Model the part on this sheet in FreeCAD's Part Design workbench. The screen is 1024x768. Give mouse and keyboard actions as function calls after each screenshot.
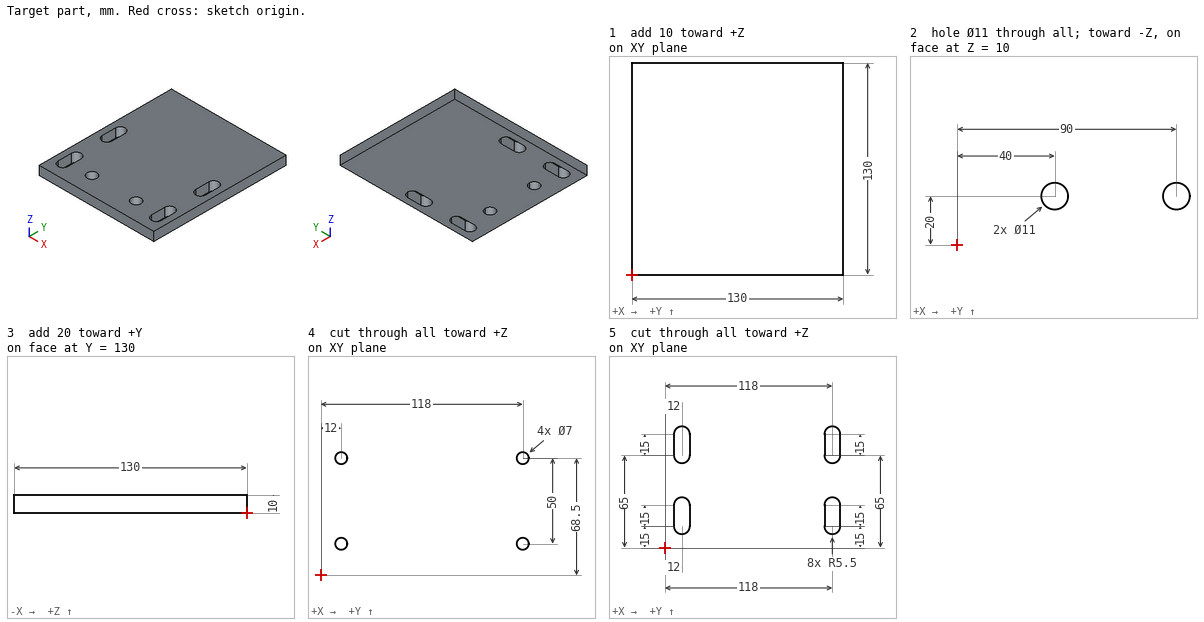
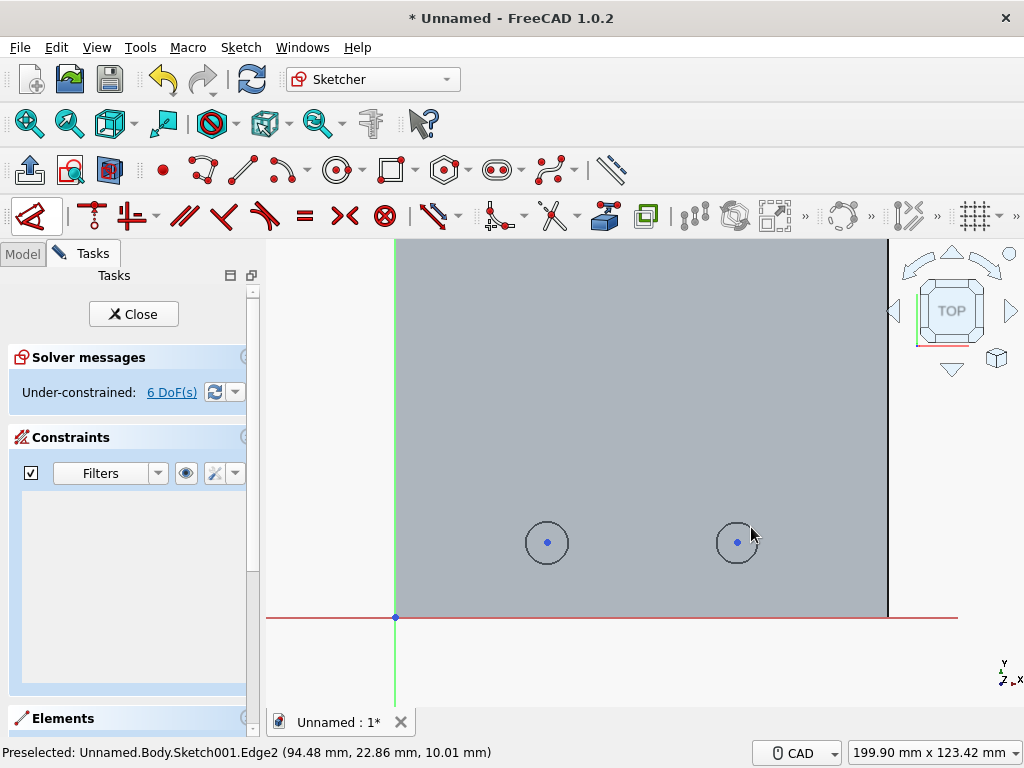
click(562, 528)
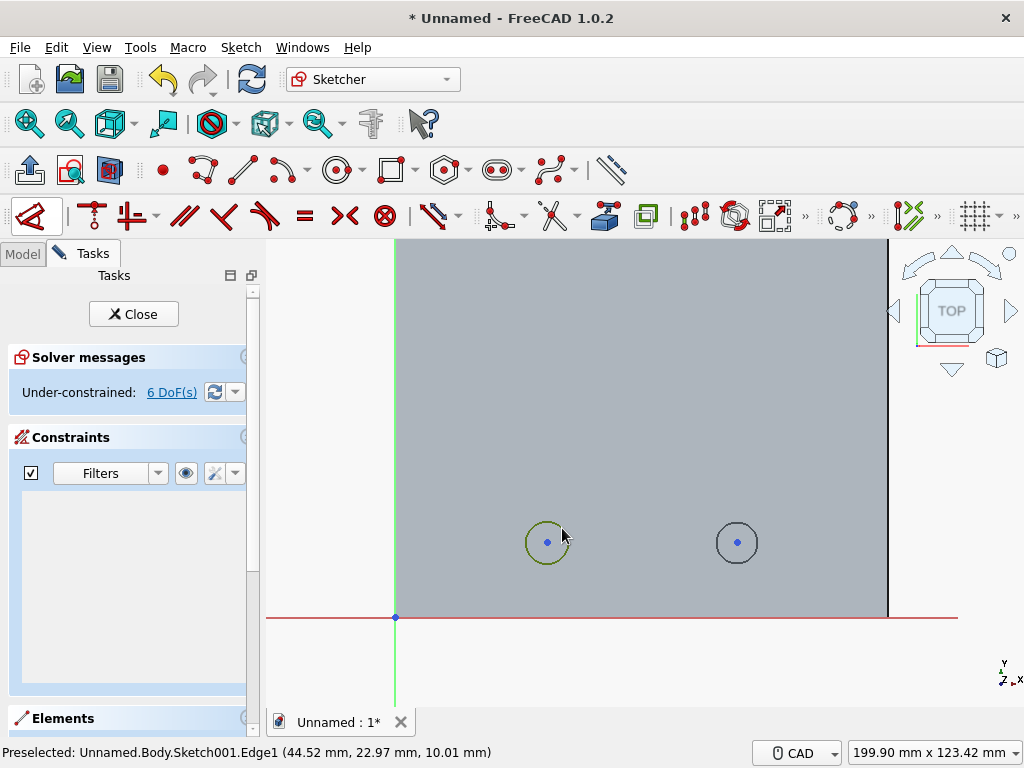
click(751, 528)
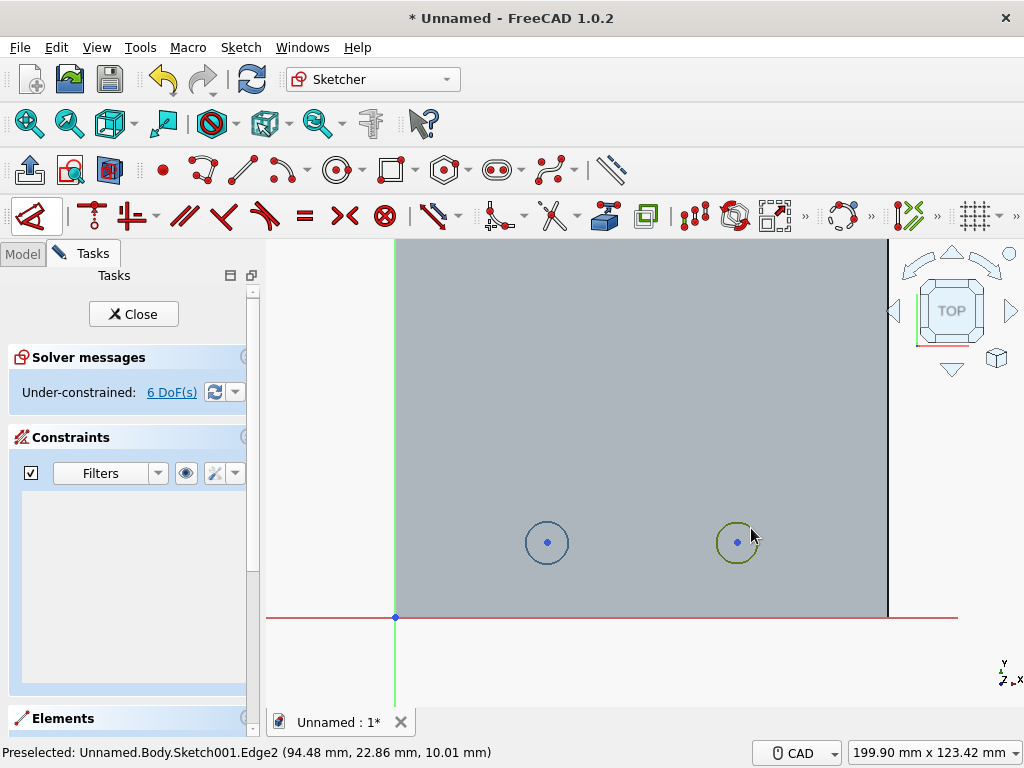
click(306, 216)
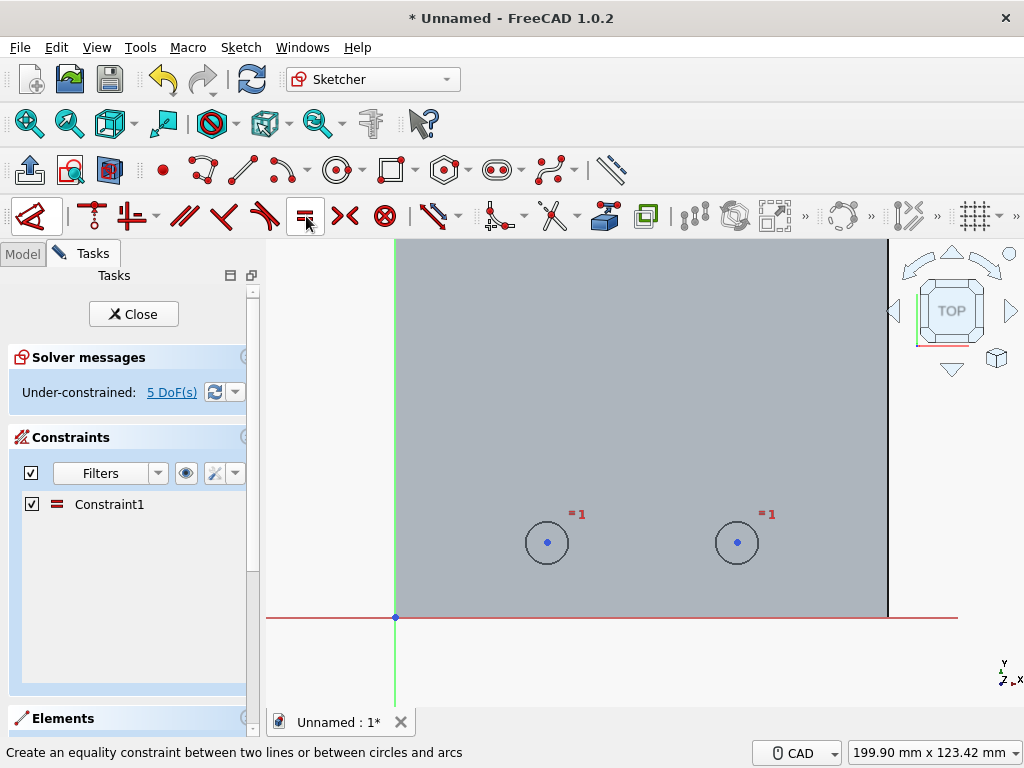
click(547, 543)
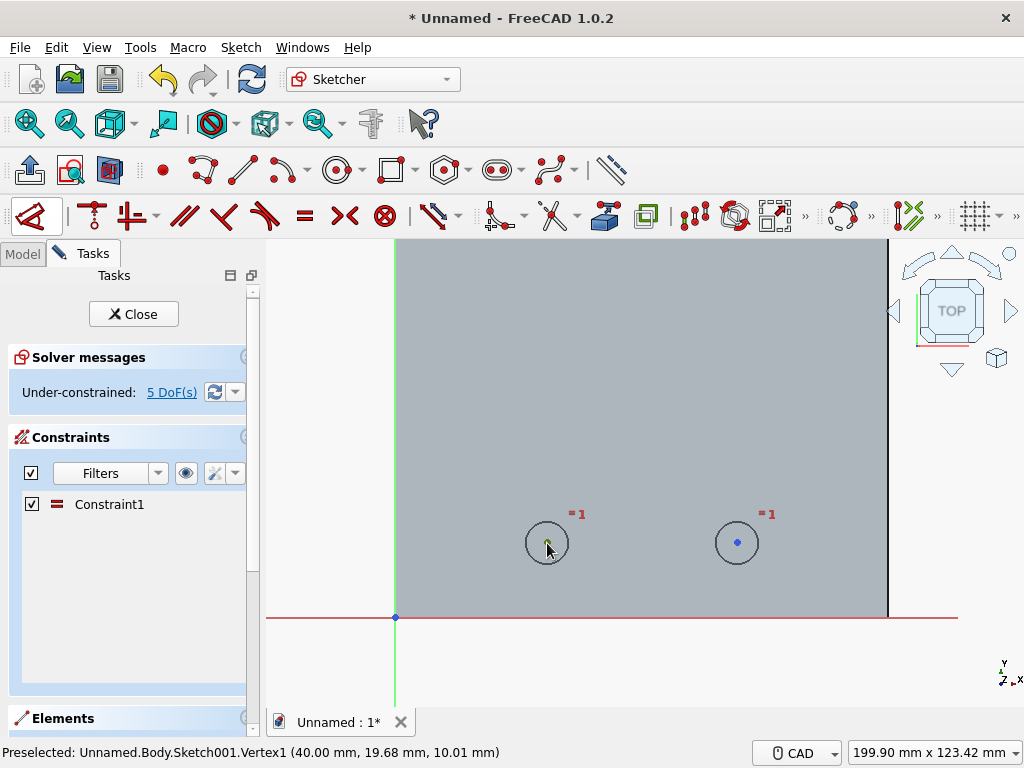
click(737, 543)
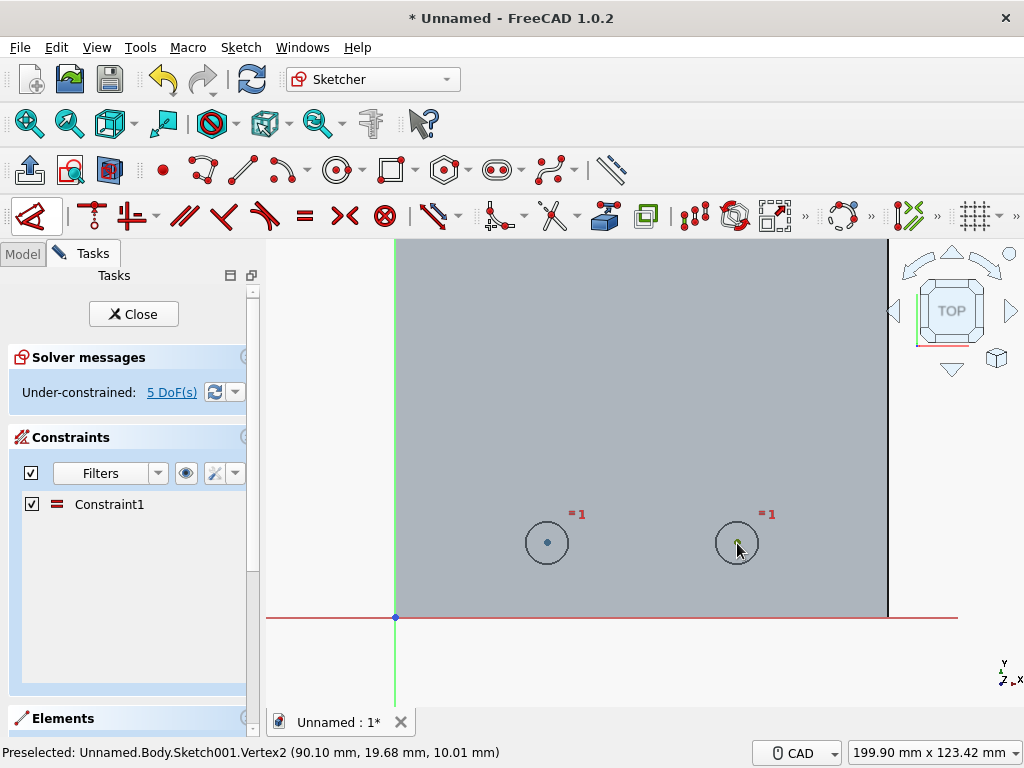
key(h)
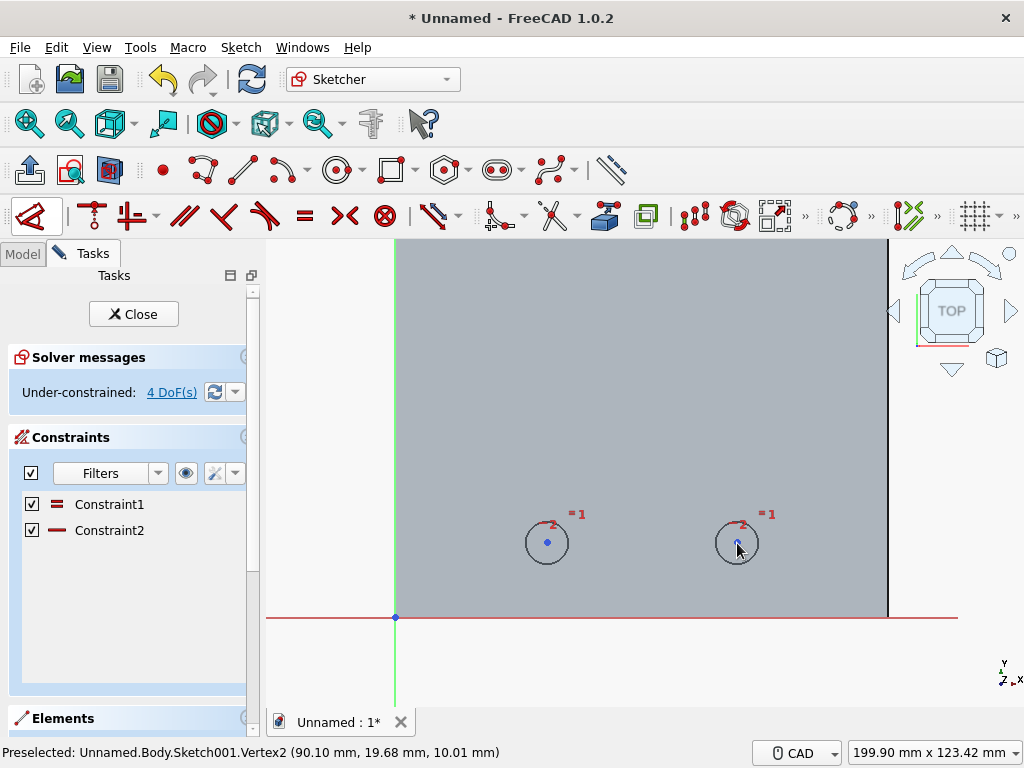
click(562, 528)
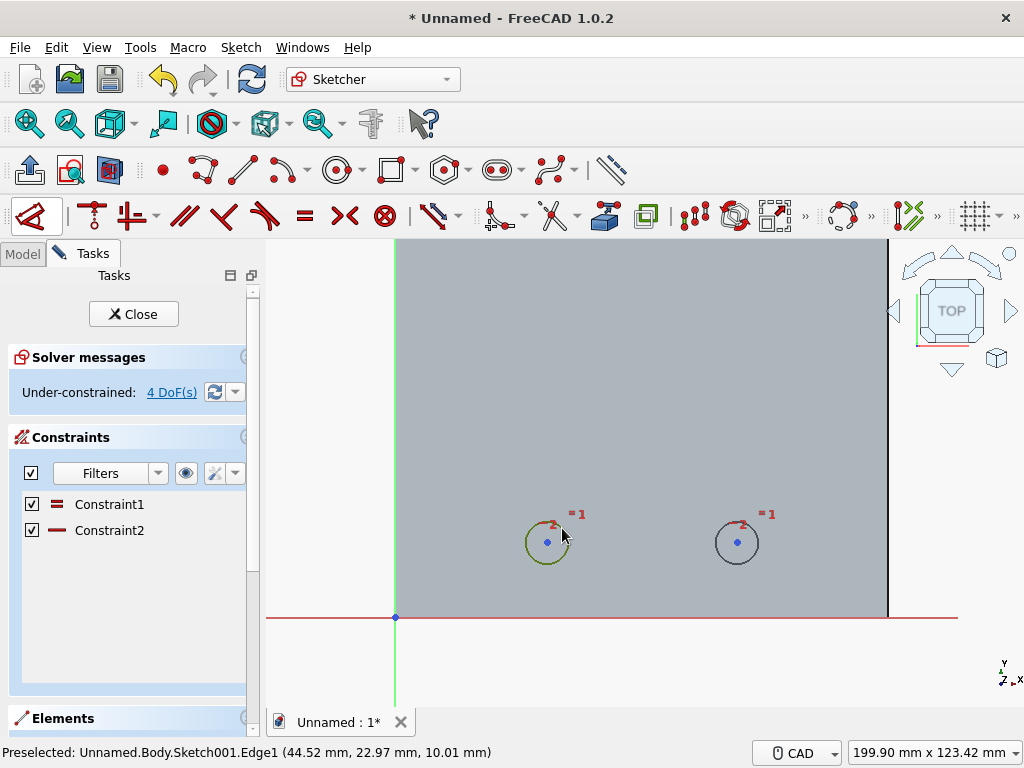
key(k)
key(o)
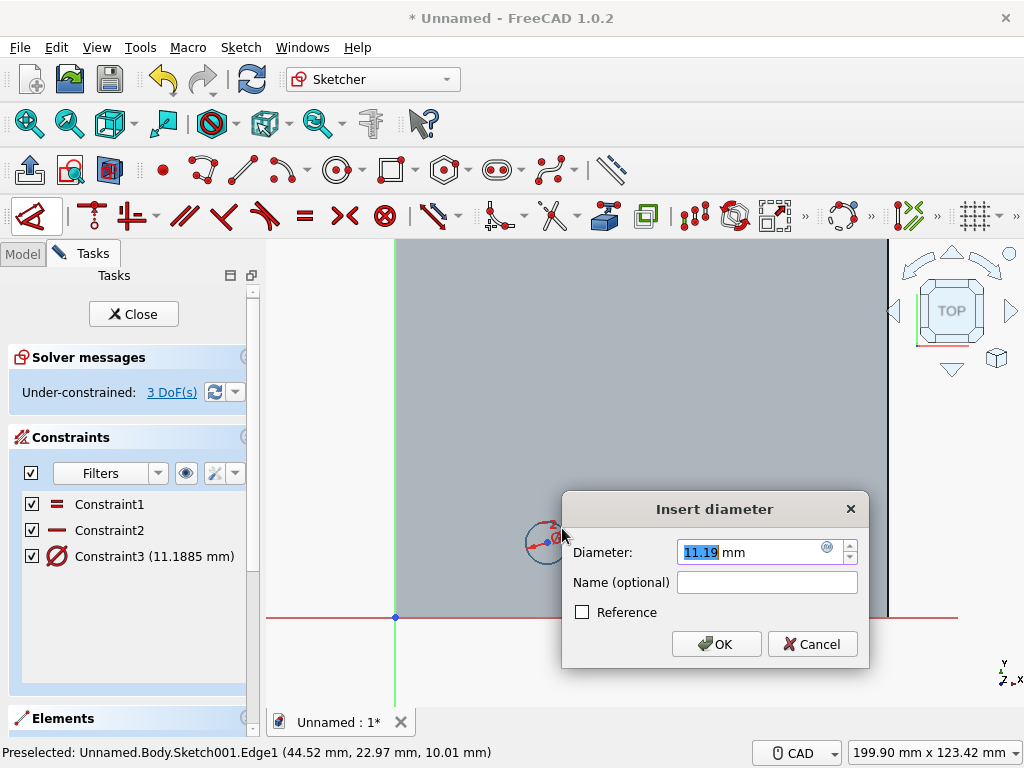
text(11)
key(Return)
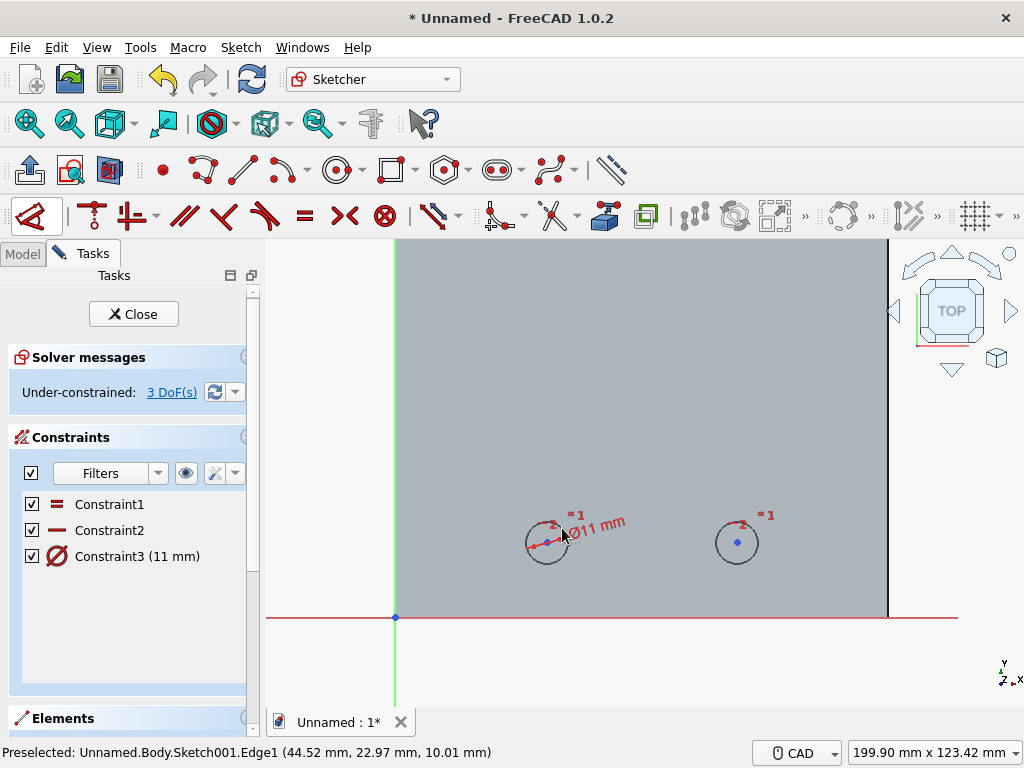
click(547, 543)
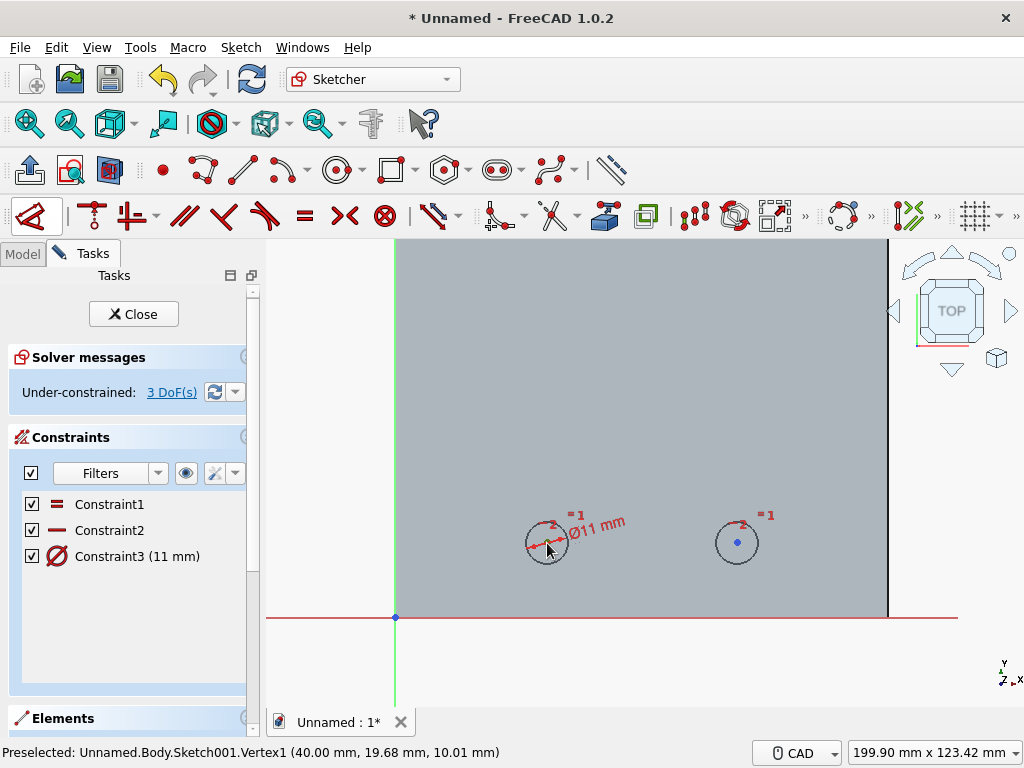
key(l)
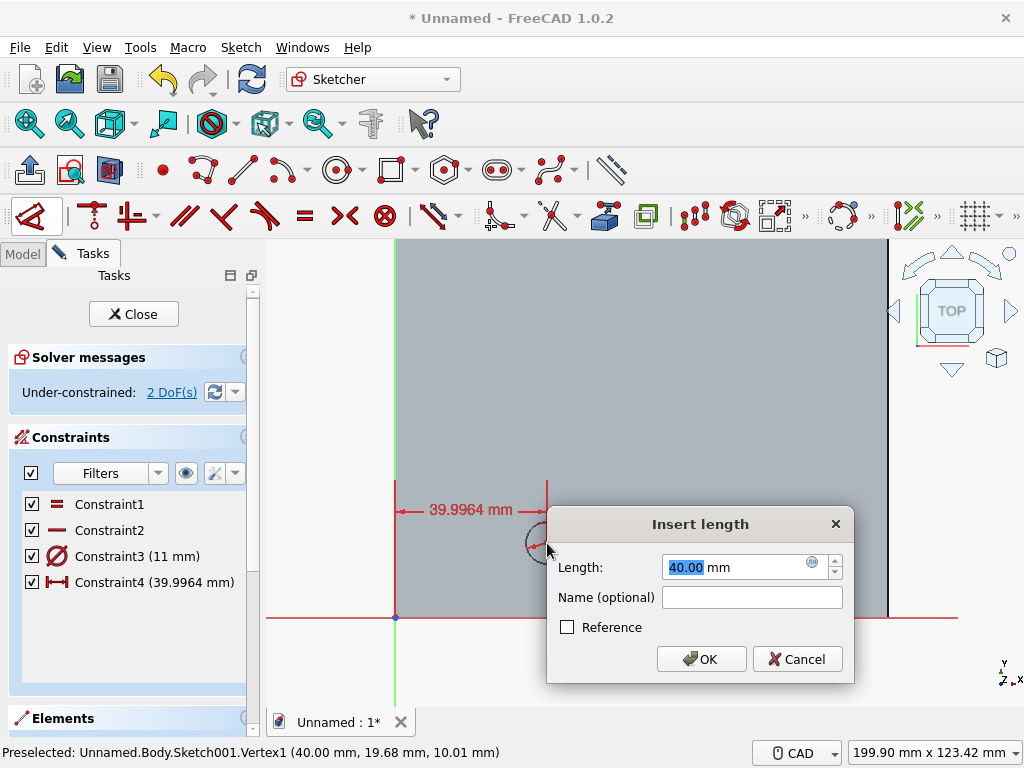
text(40)
key(Return)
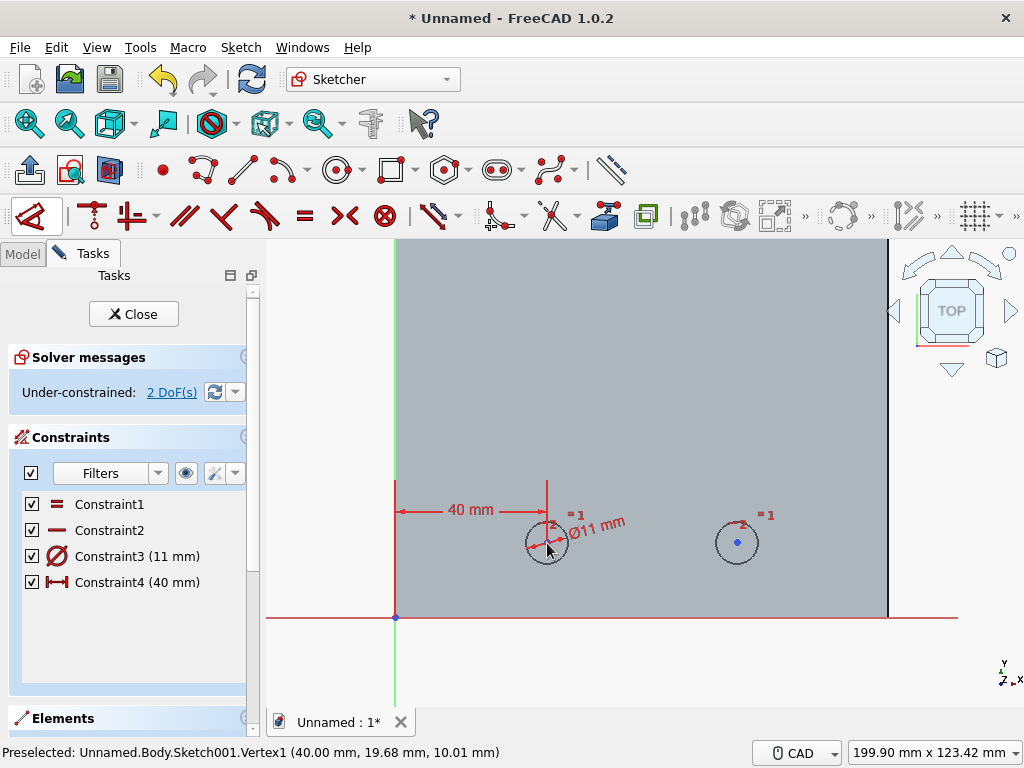
click(547, 543)